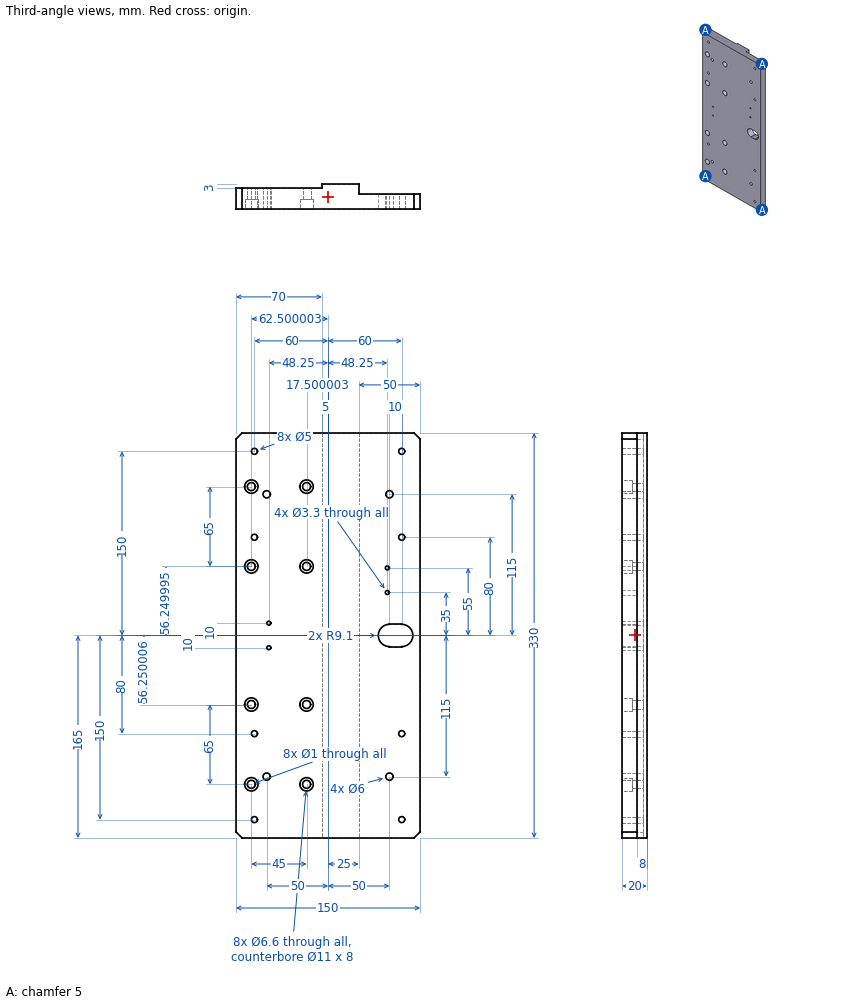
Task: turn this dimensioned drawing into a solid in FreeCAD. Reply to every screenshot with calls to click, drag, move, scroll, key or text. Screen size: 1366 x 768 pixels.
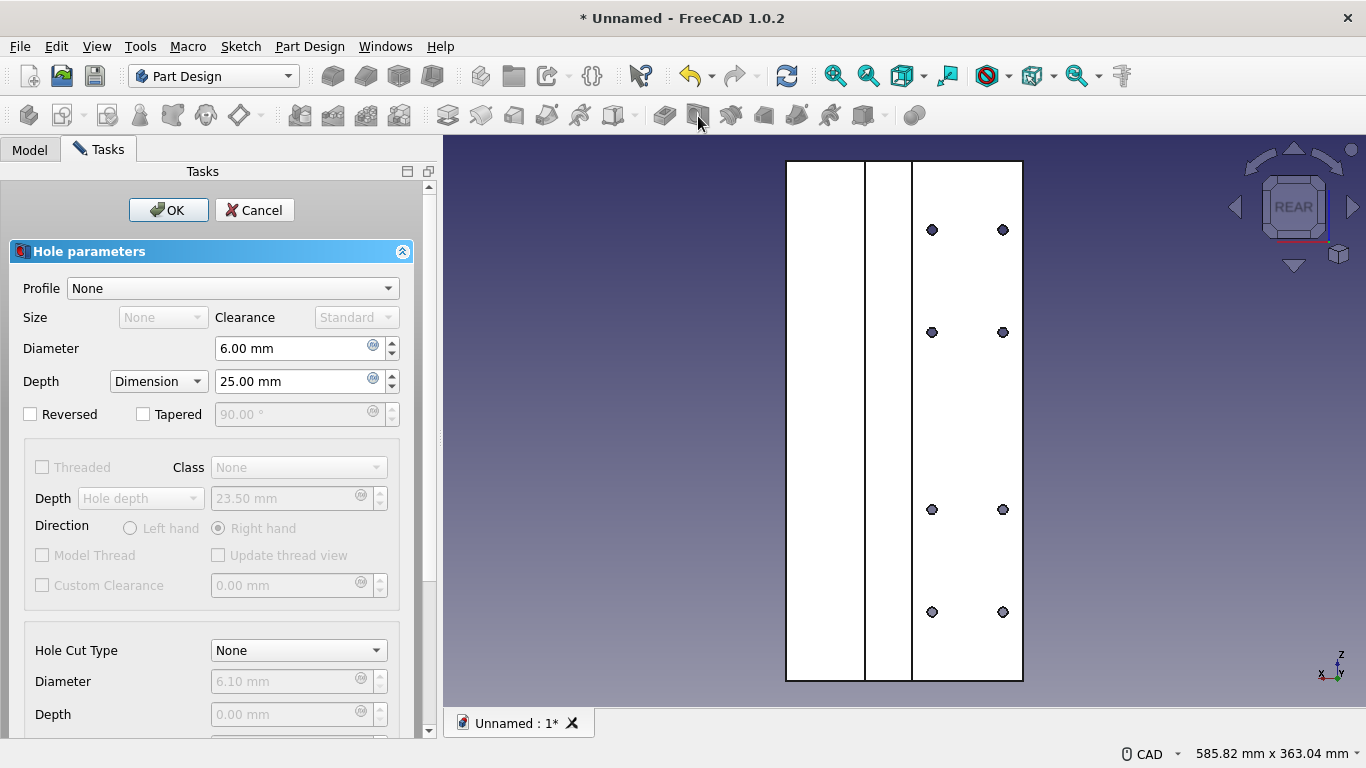
triple_click(300, 348)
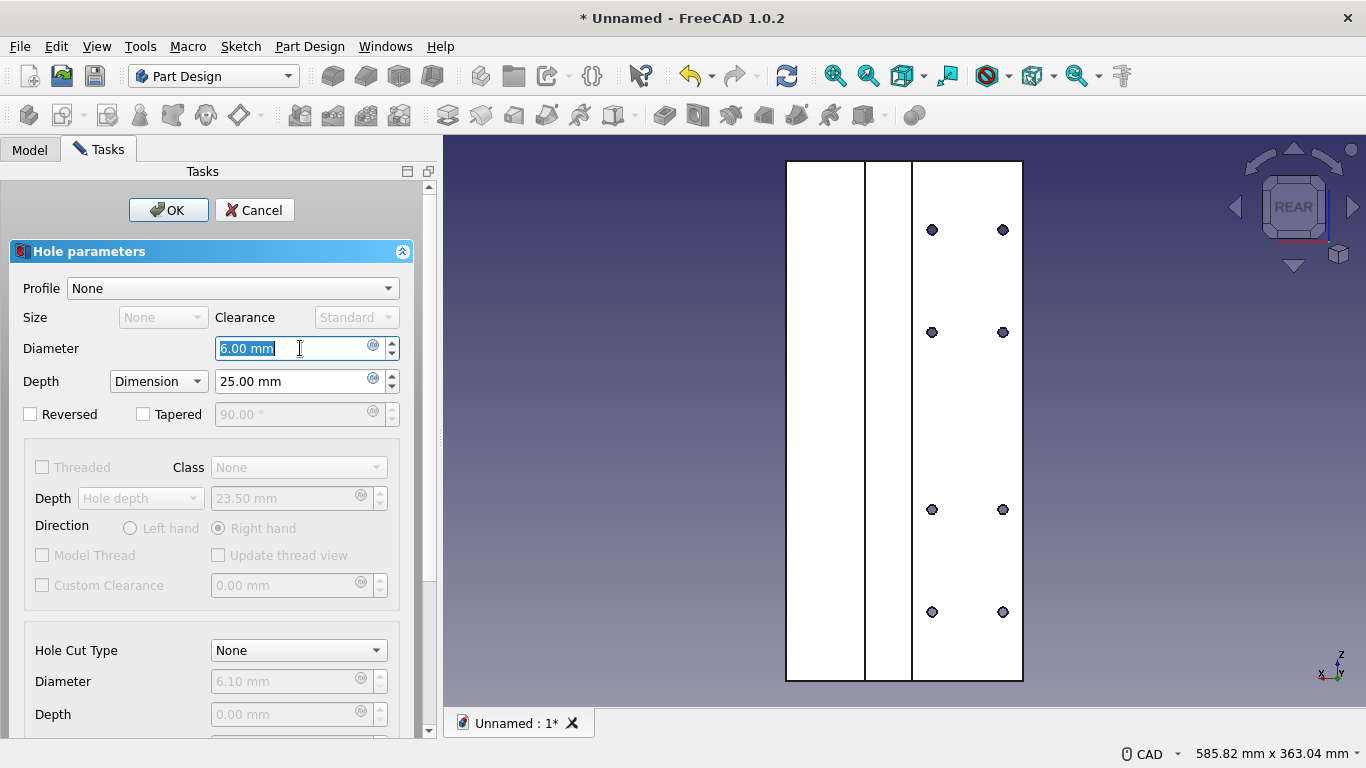
text(1)
key(Tab)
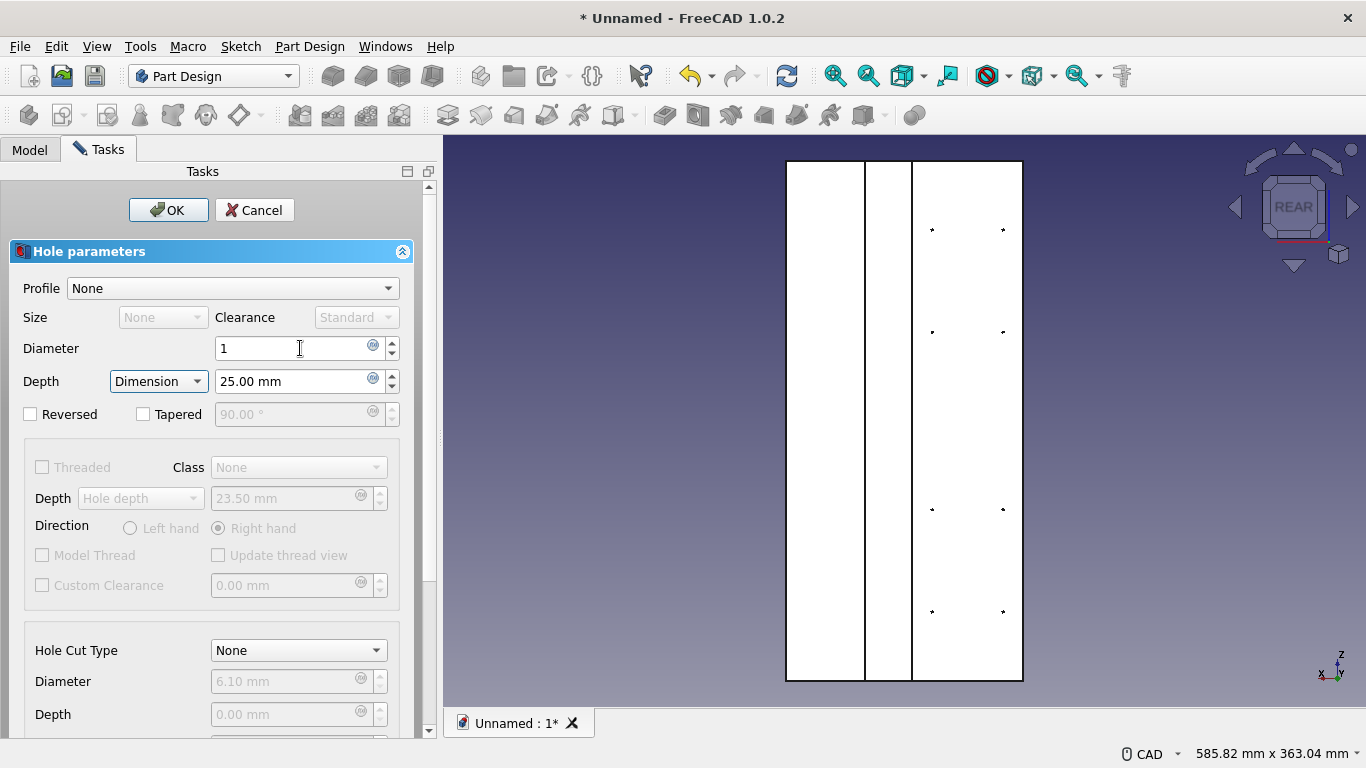
click(160, 382)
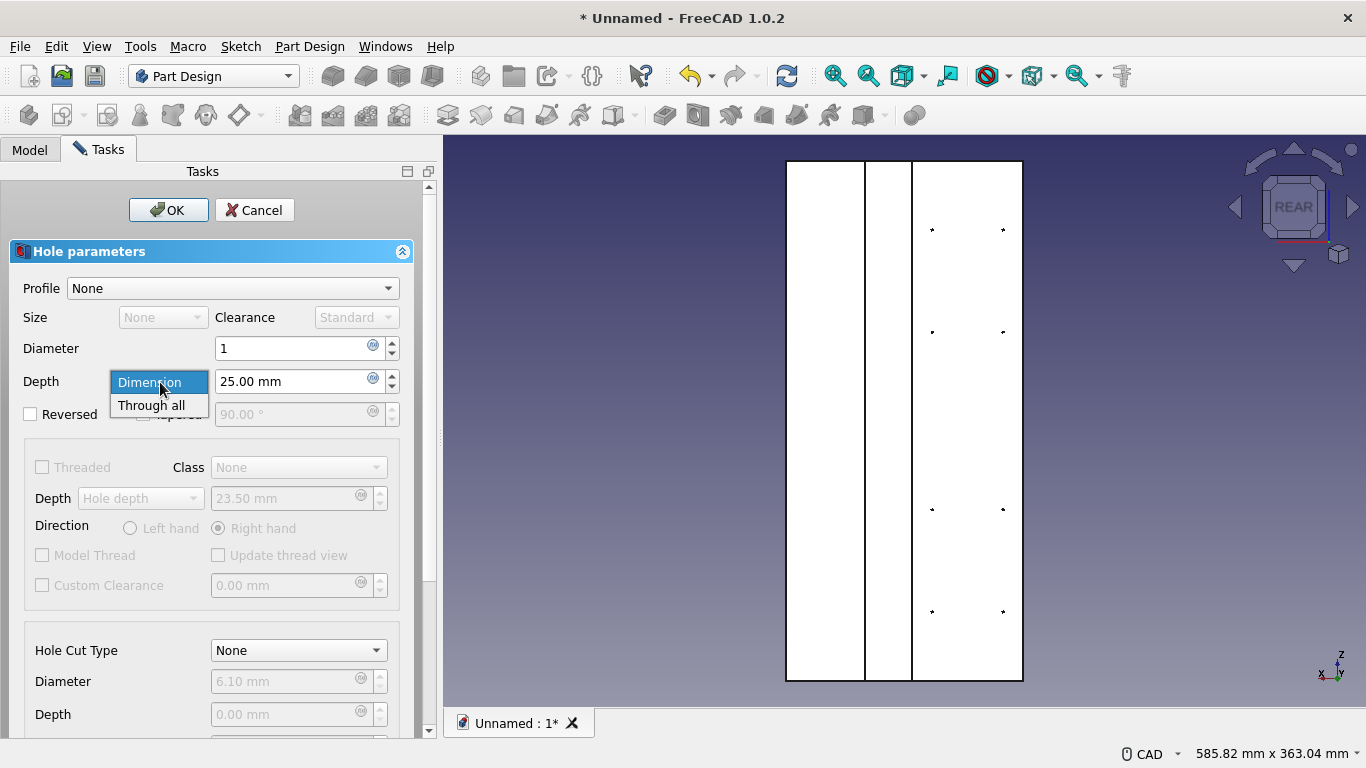
click(158, 406)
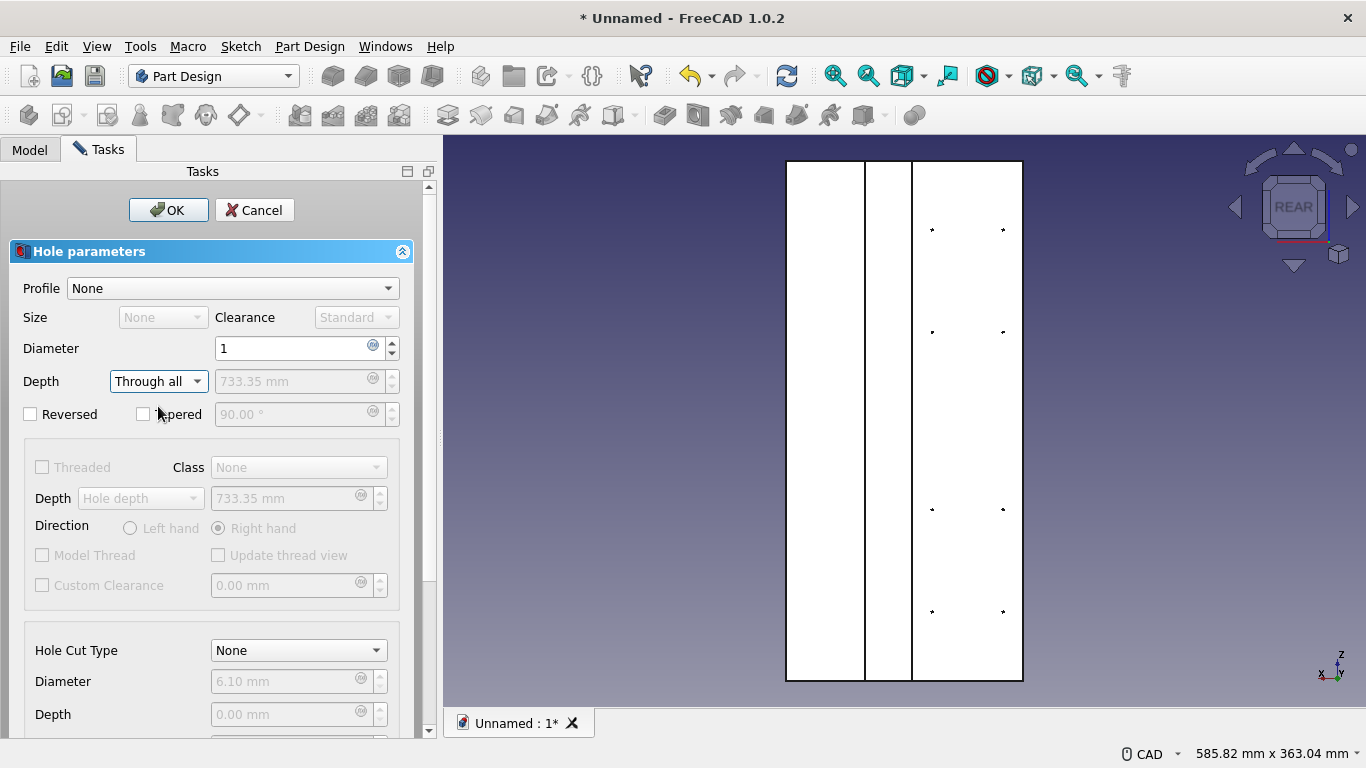
click(169, 210)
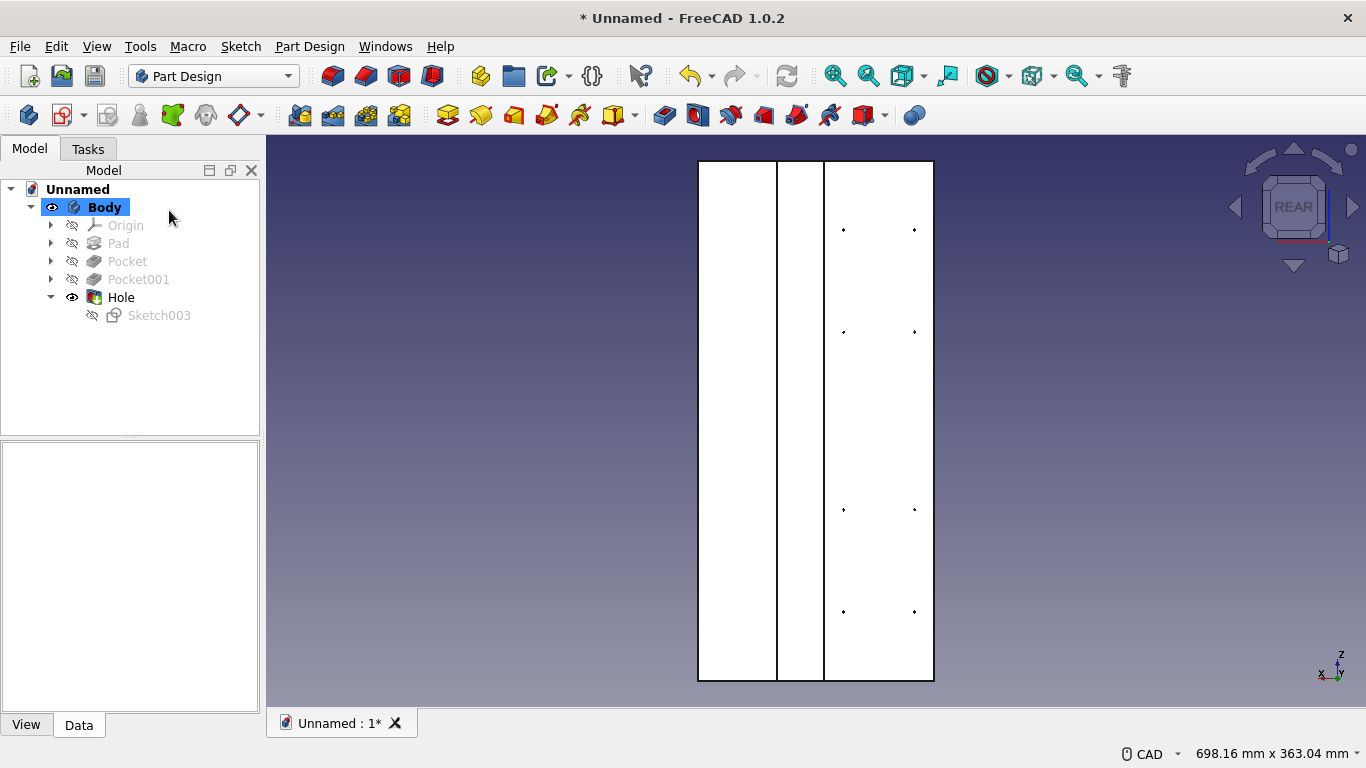
key(0)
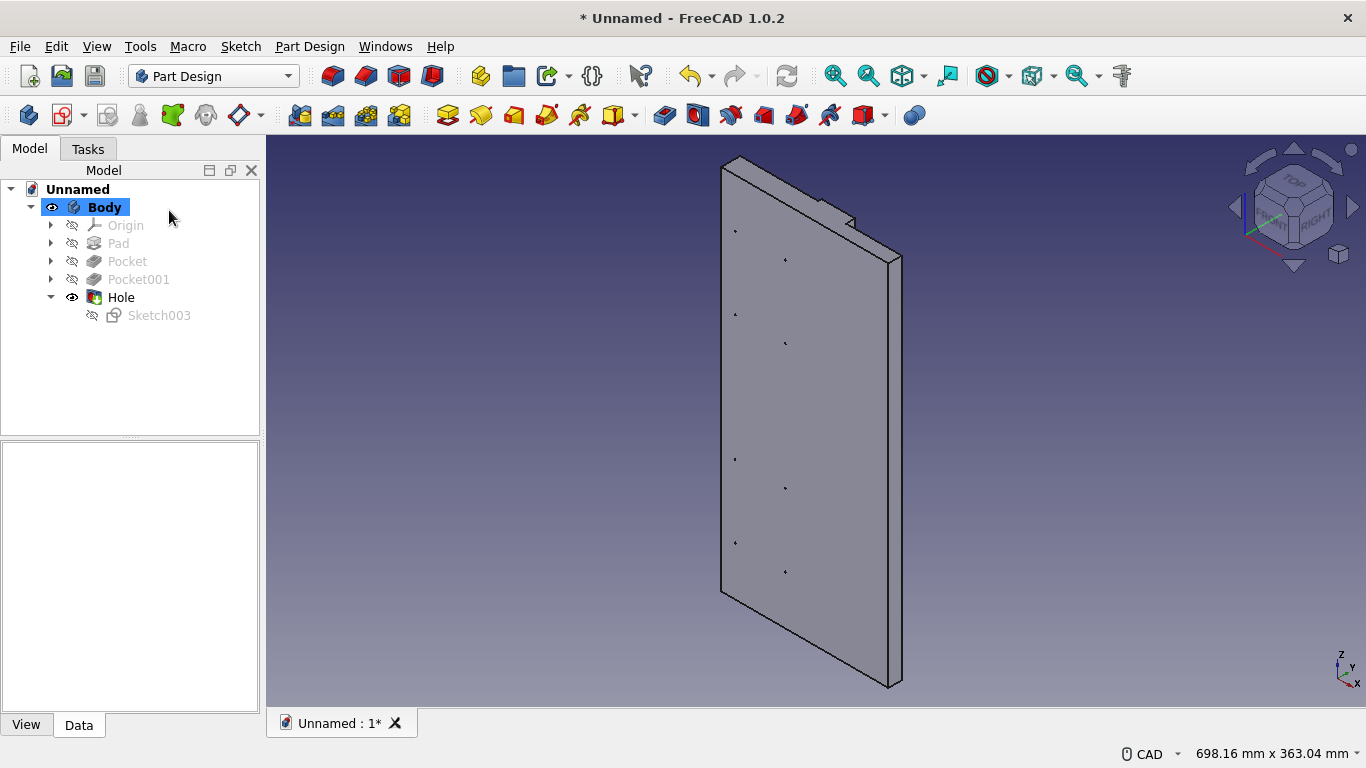
click(805, 426)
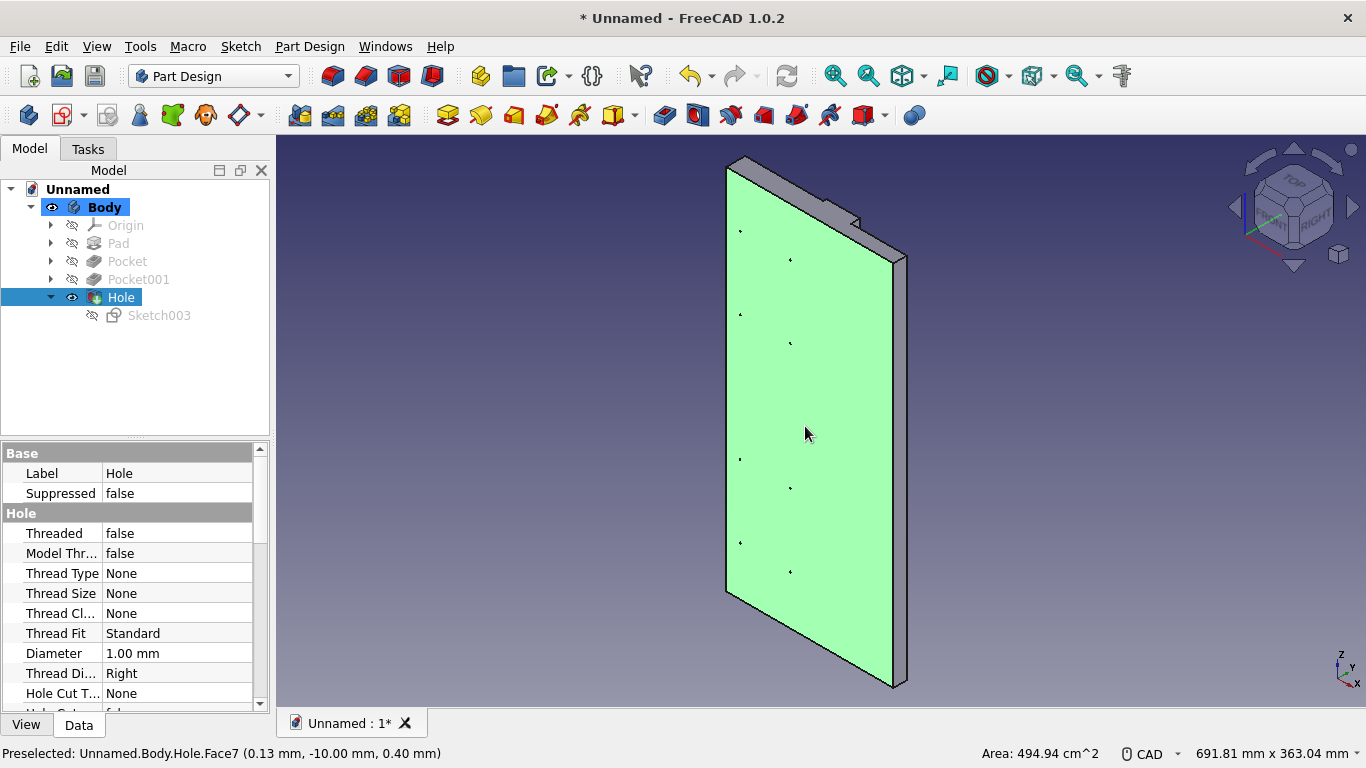
click(62, 116)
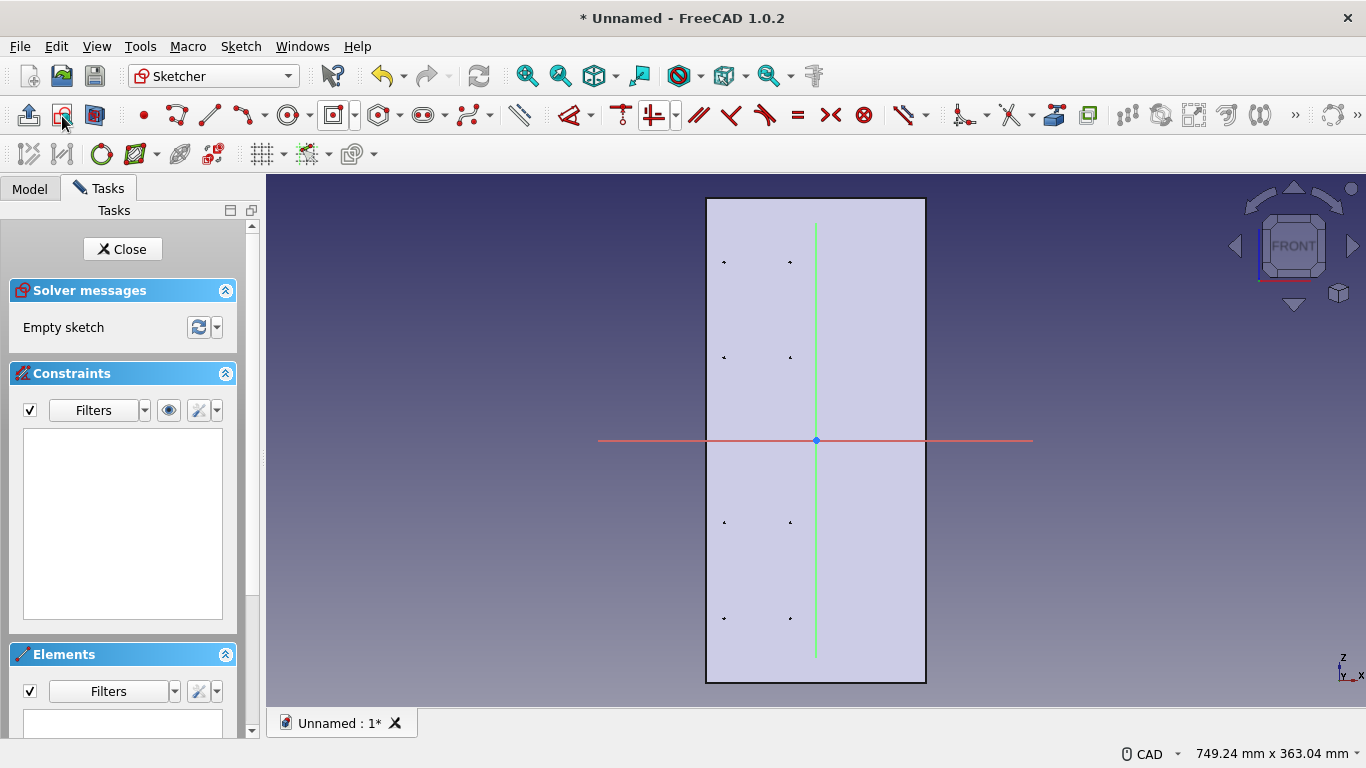
click(288, 116)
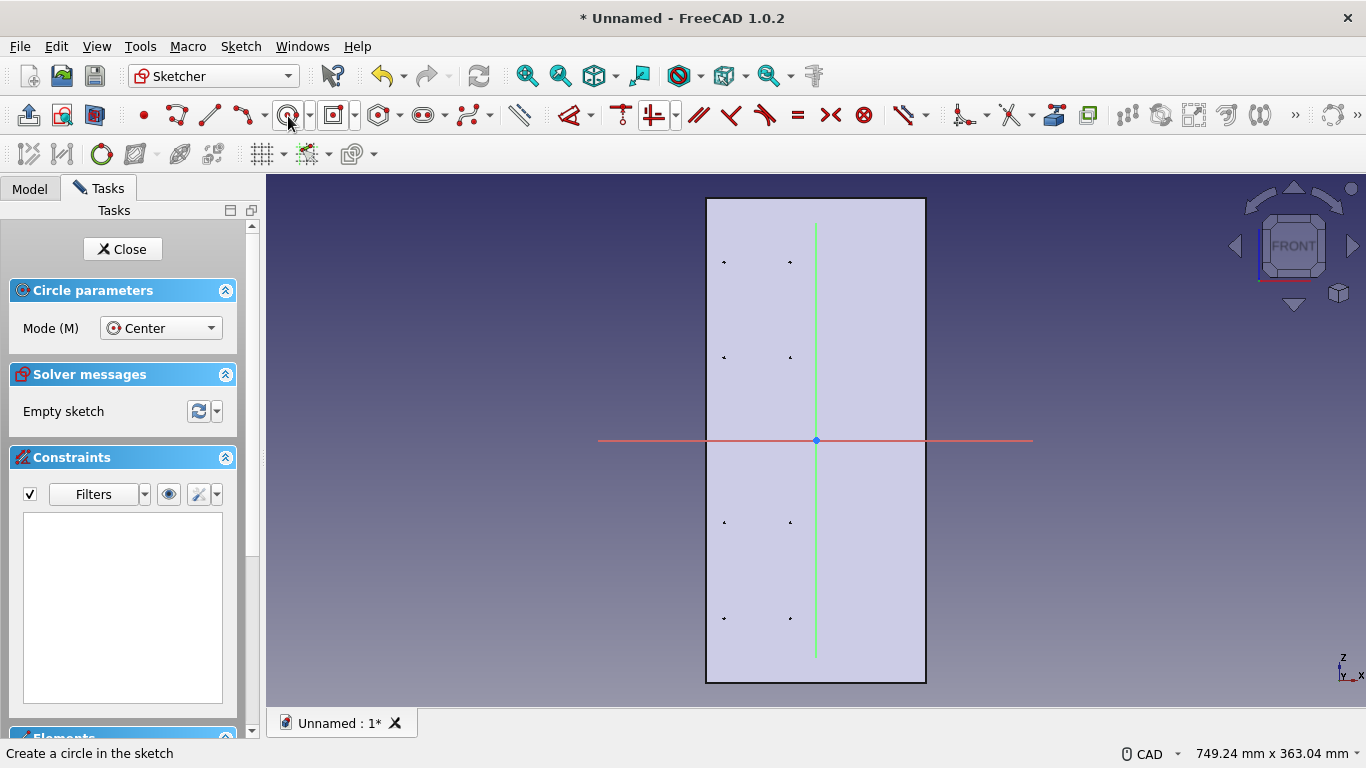
scroll(790, 619, up, 8)